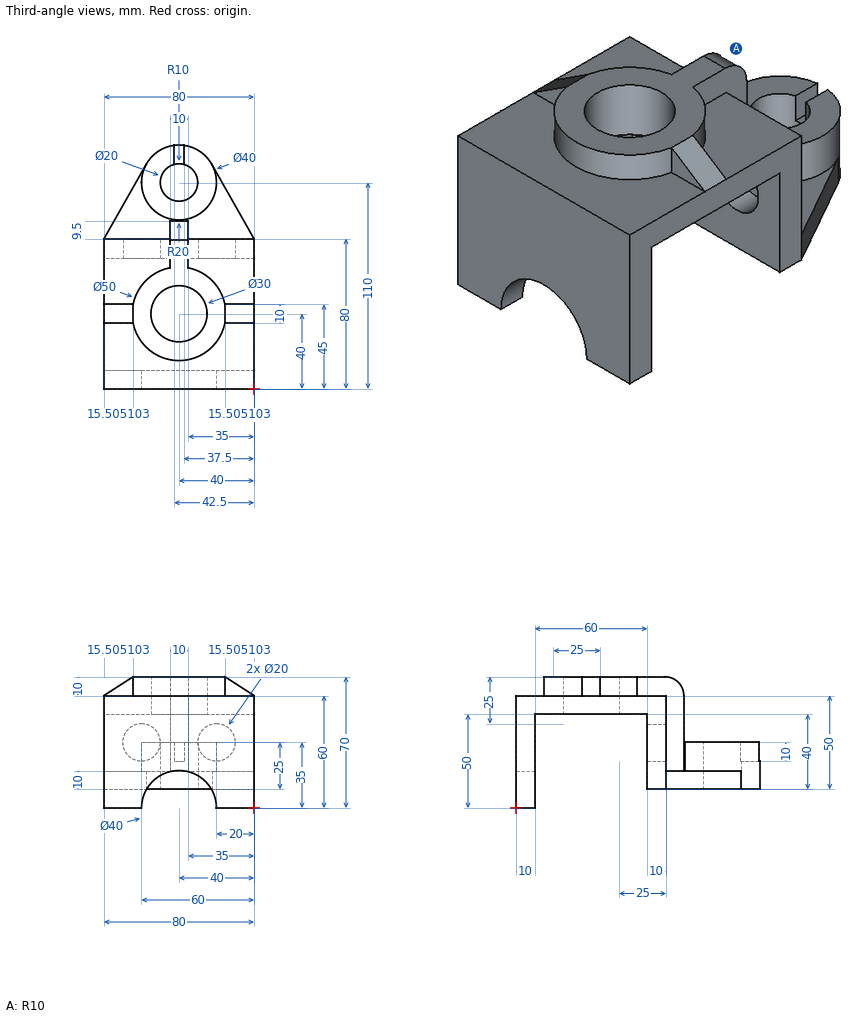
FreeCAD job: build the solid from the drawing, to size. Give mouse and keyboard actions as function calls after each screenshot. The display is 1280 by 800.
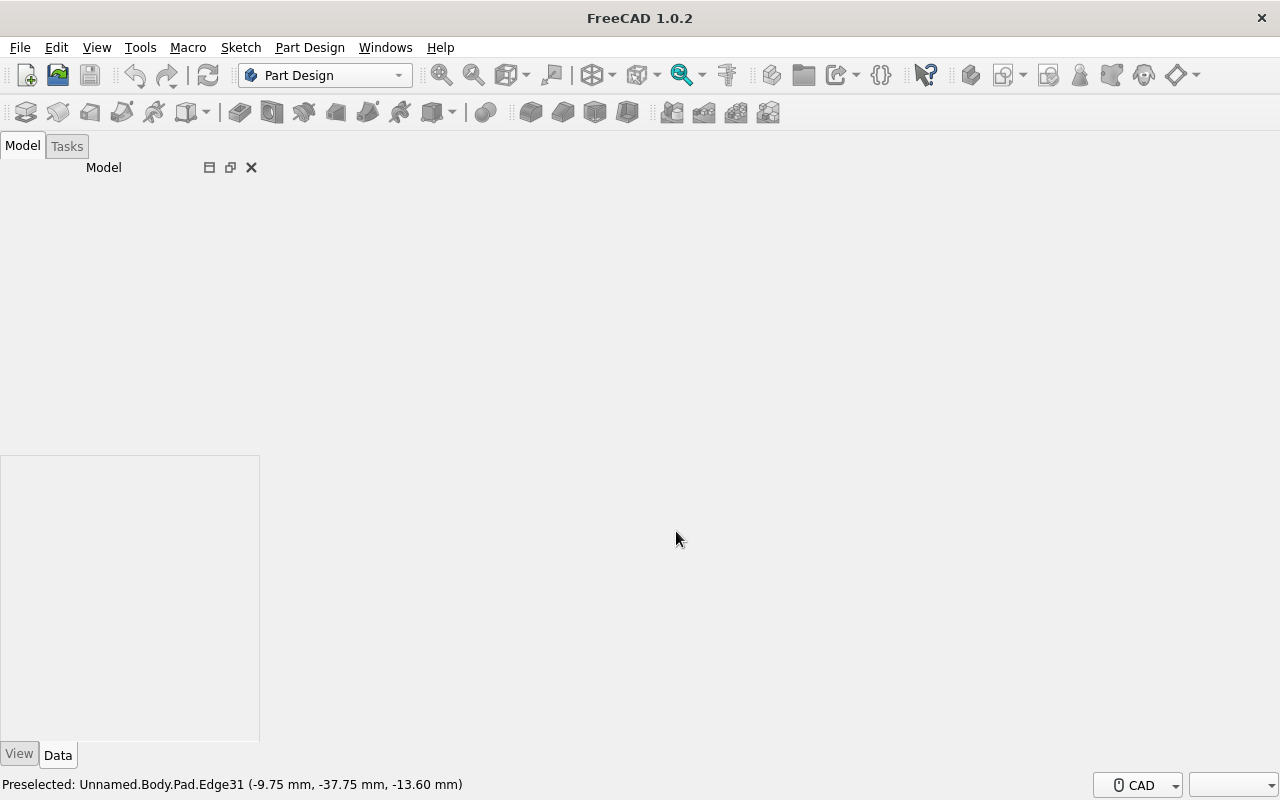
click(26, 76)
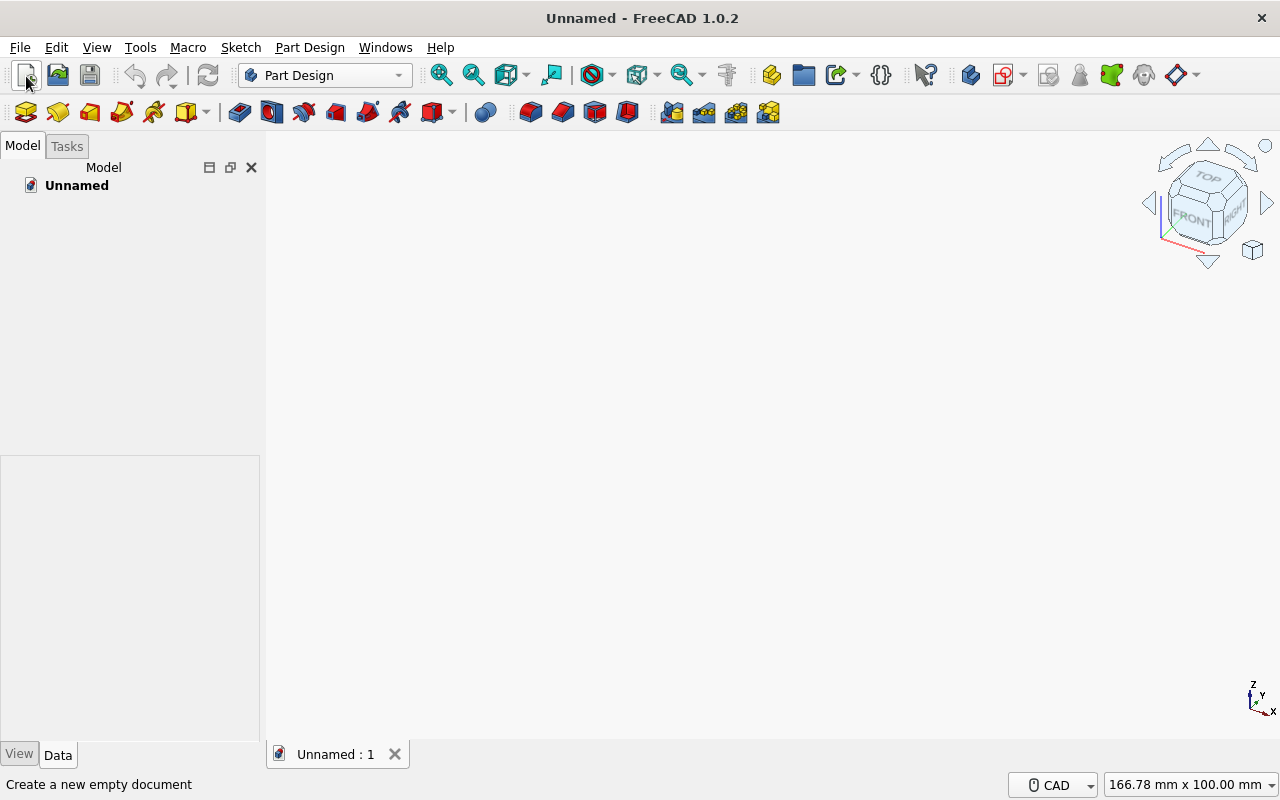
click(1004, 76)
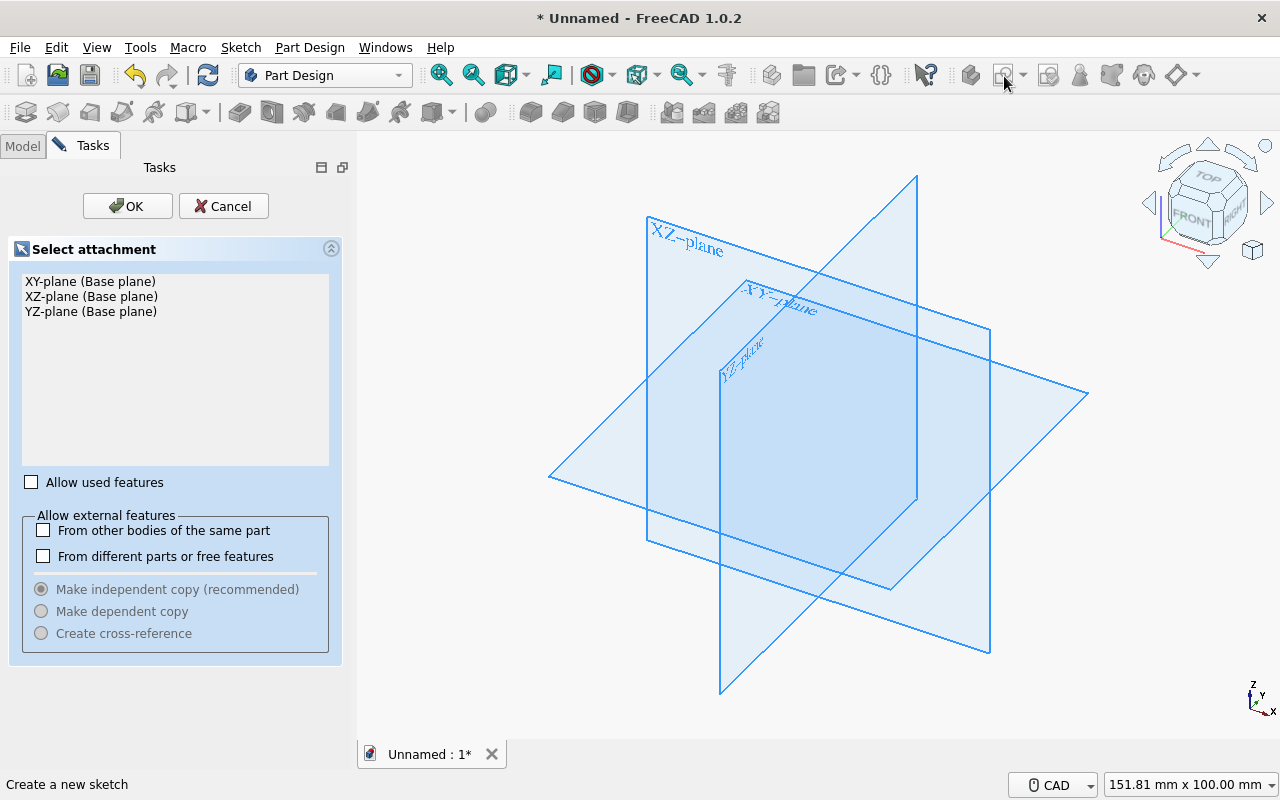
click(82, 312)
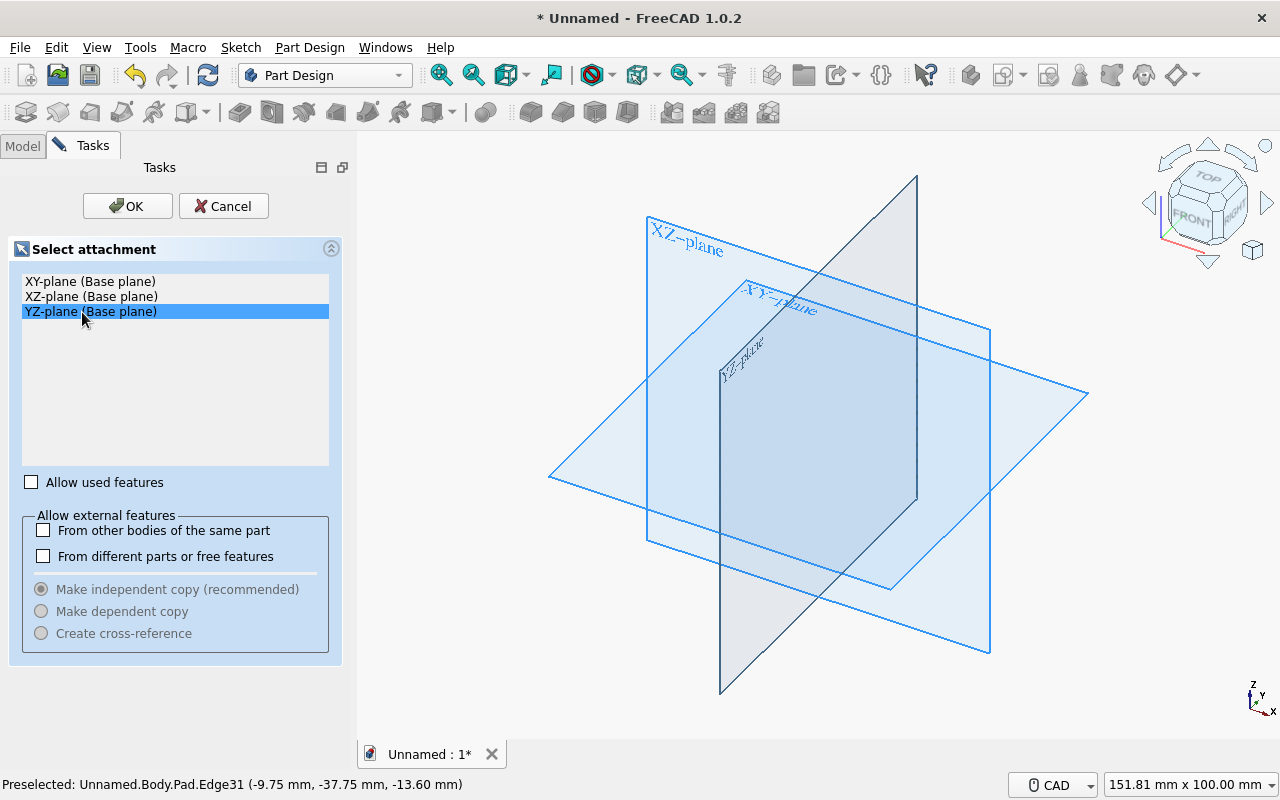
click(128, 206)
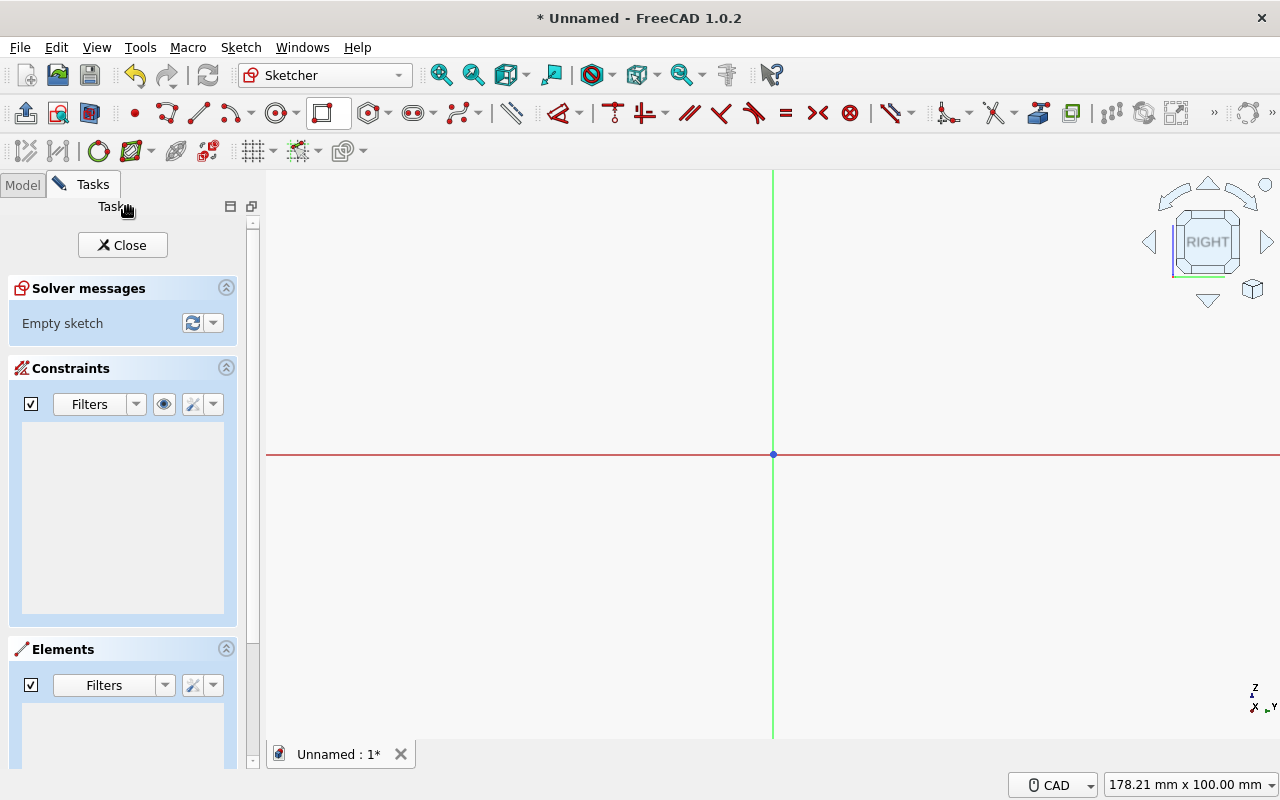
scroll(294, 711, down, 2)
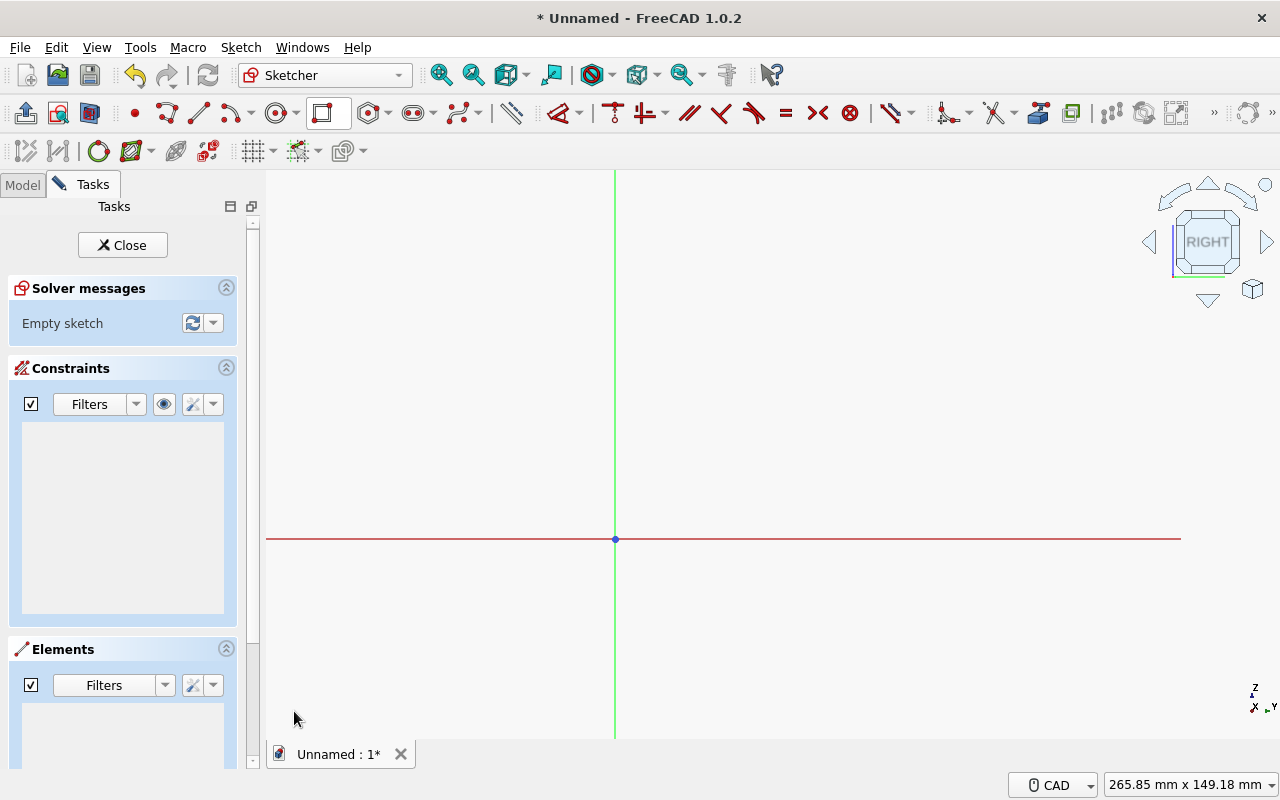
scroll(896, 365, up, 2)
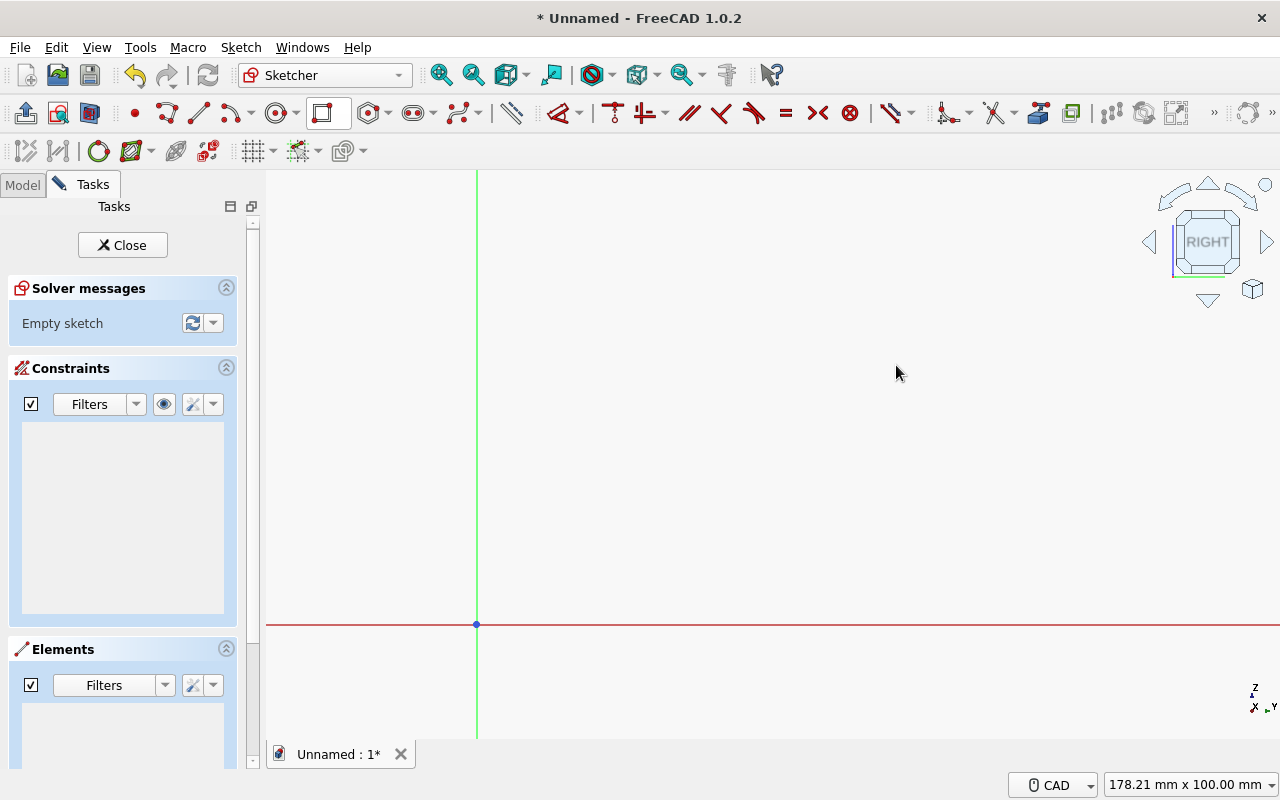
click(168, 114)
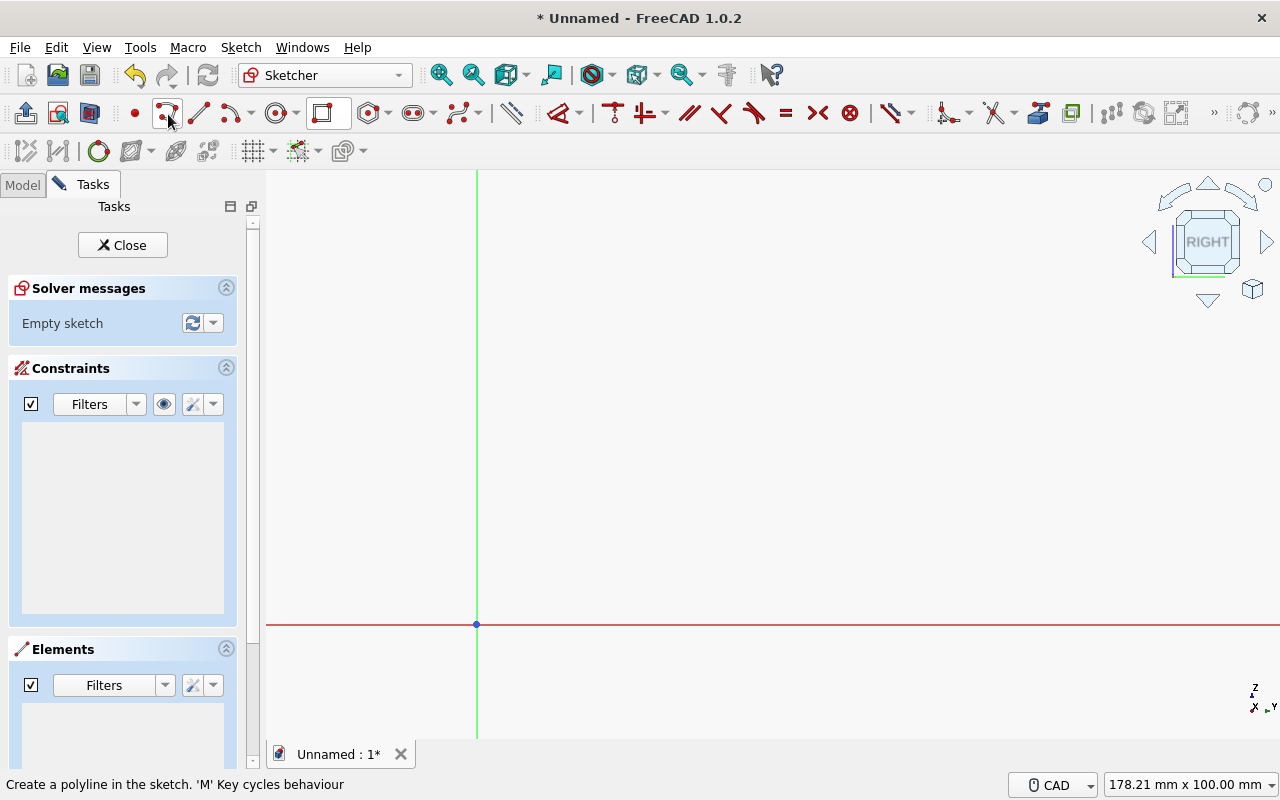
click(477, 625)
click(534, 616)
click(534, 340)
click(875, 340)
click(875, 568)
click(932, 568)
click(932, 284)
click(486, 284)
click(477, 625)
key(Escape)
key(Escape)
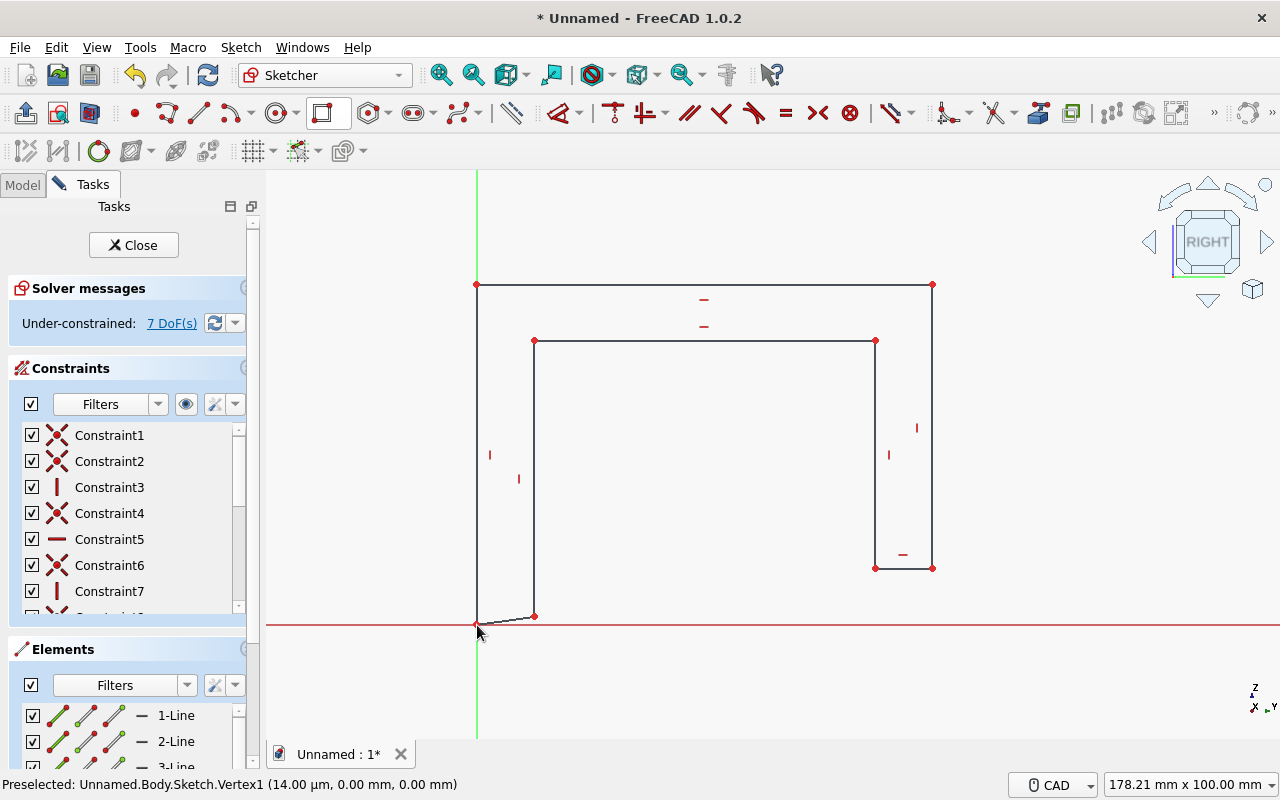
click(494, 623)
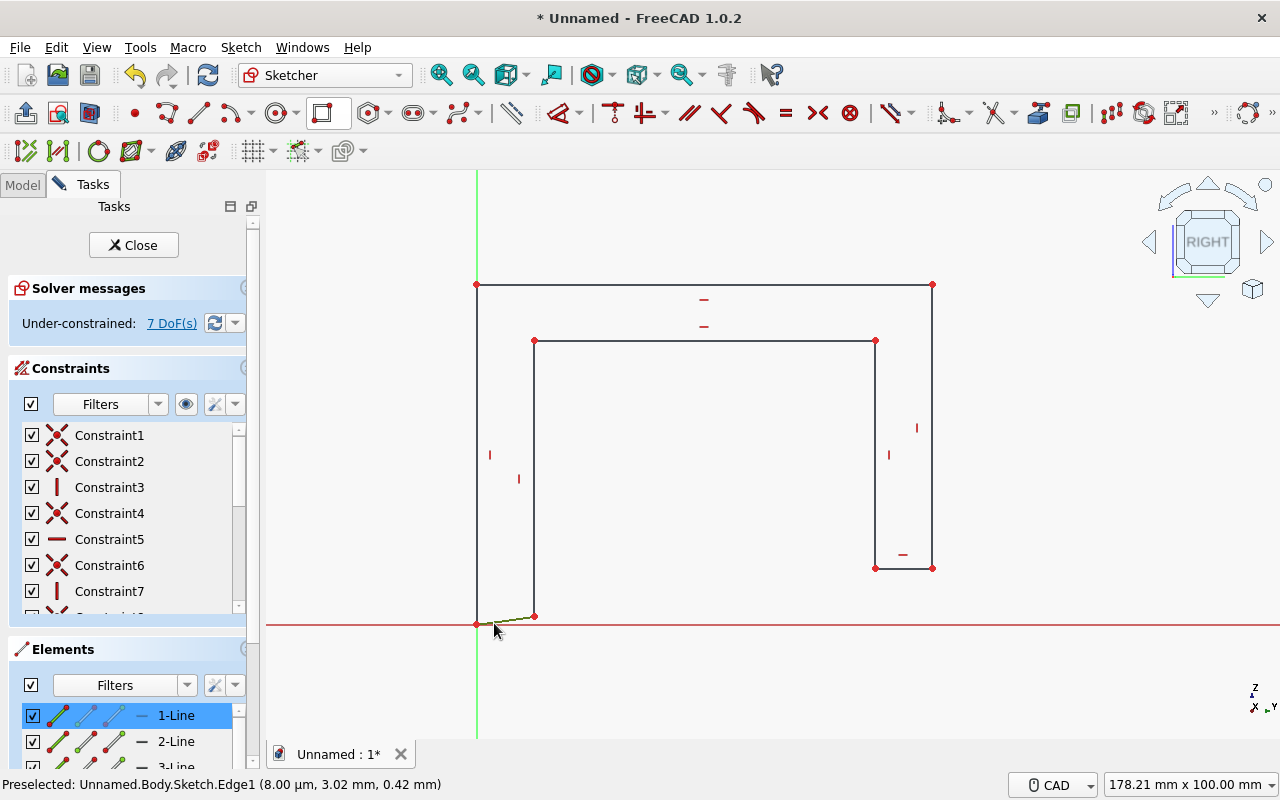
click(668, 114)